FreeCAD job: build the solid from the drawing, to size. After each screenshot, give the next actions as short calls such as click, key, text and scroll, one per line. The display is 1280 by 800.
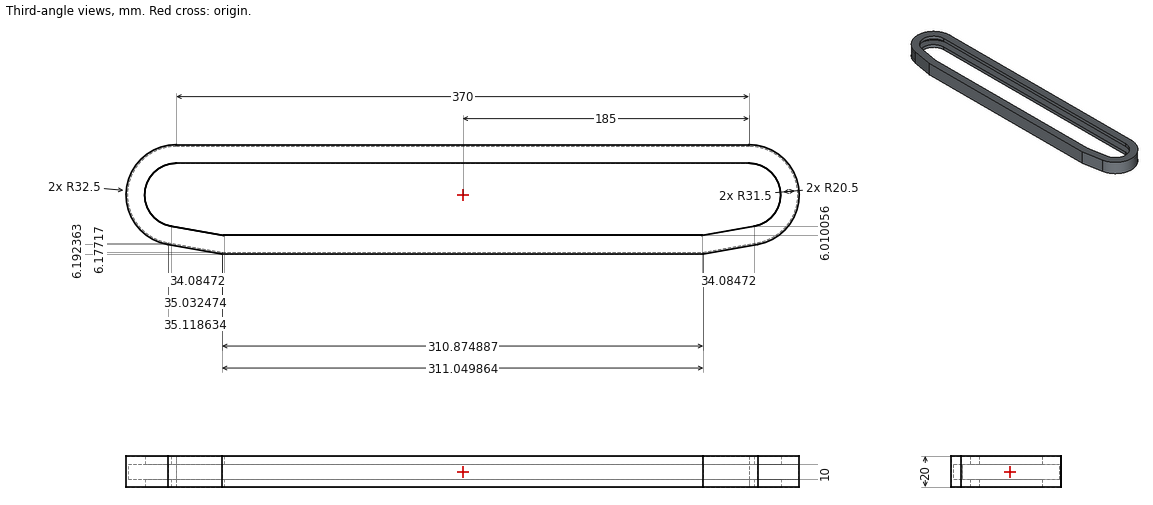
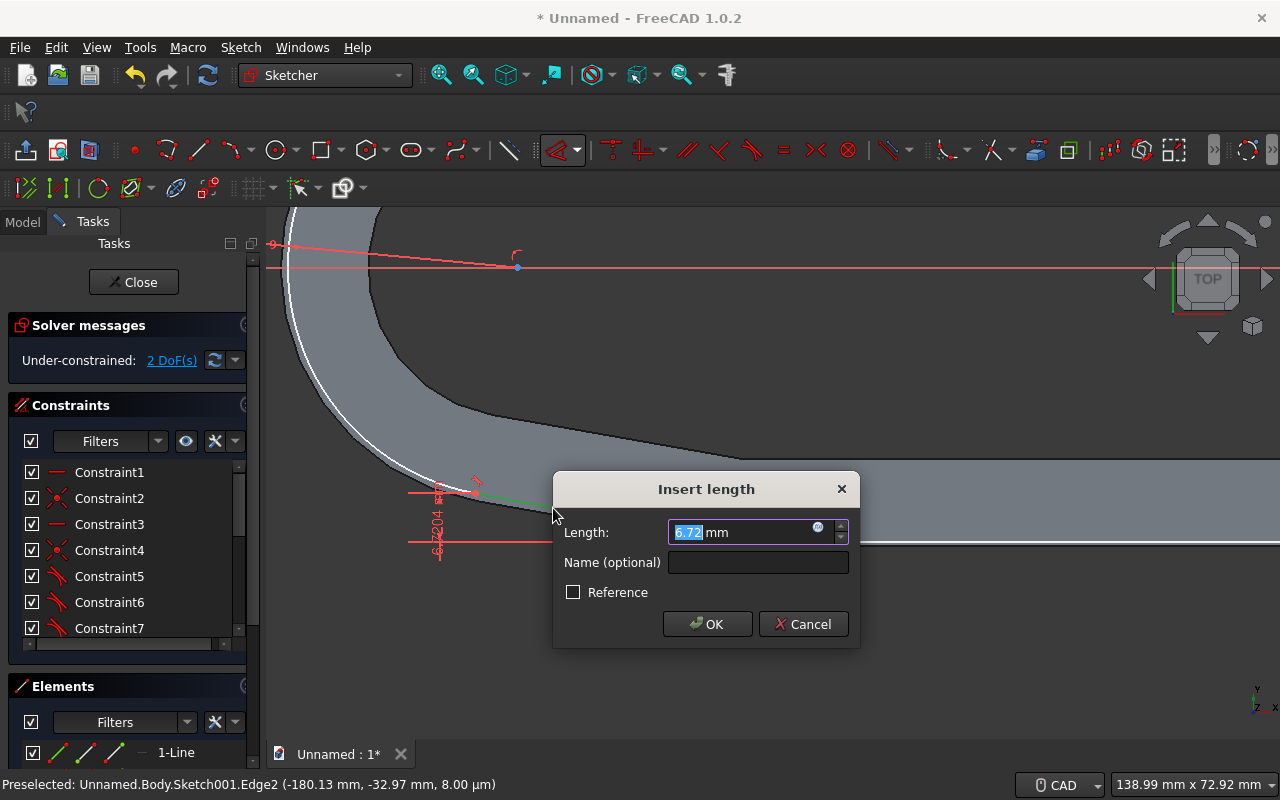
text(6.17717)
key(Return)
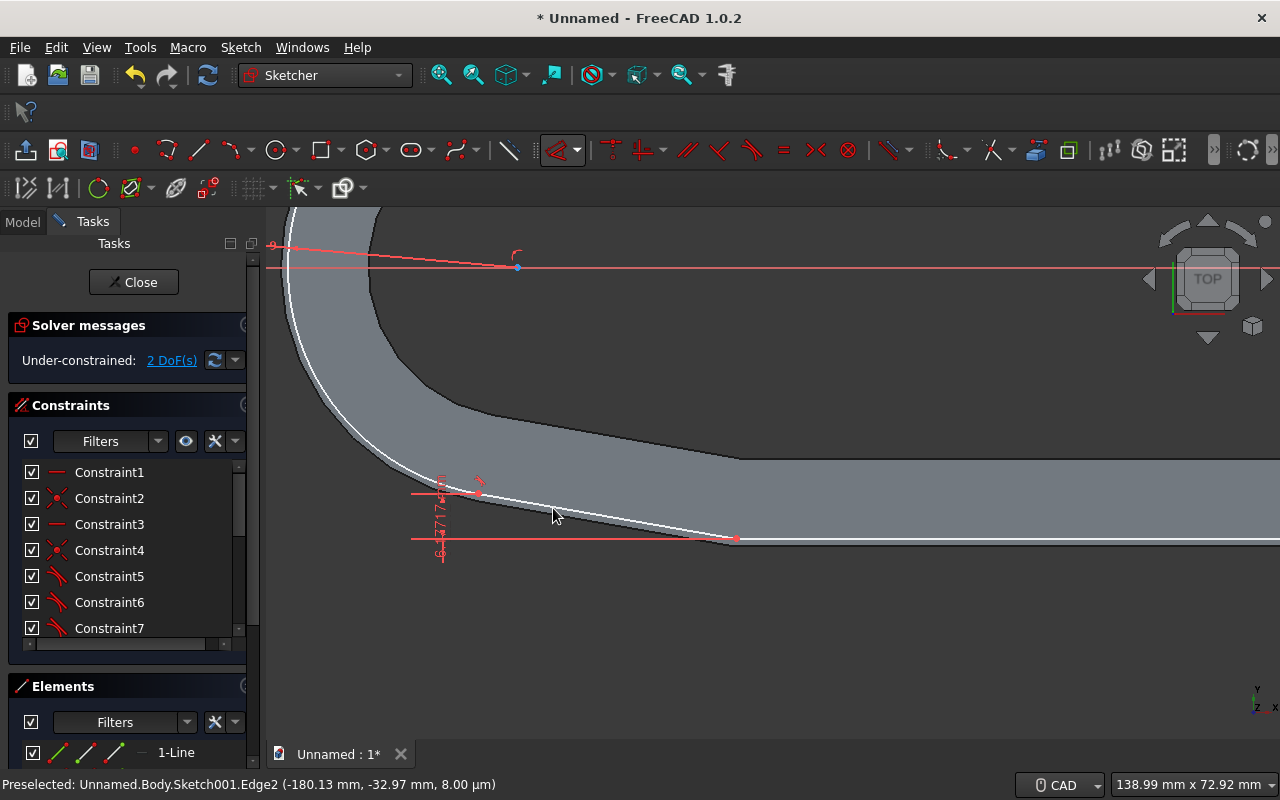
scroll(410, 520, down, 8)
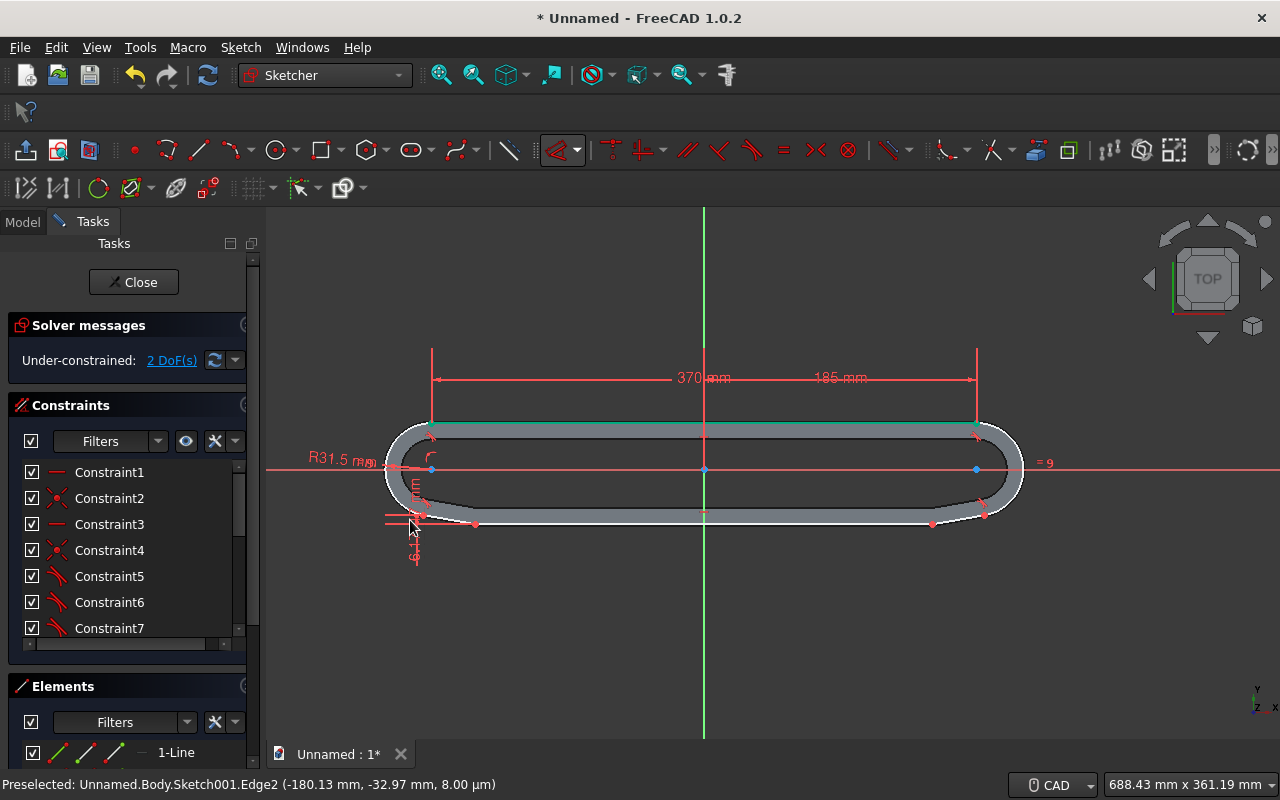
click(613, 524)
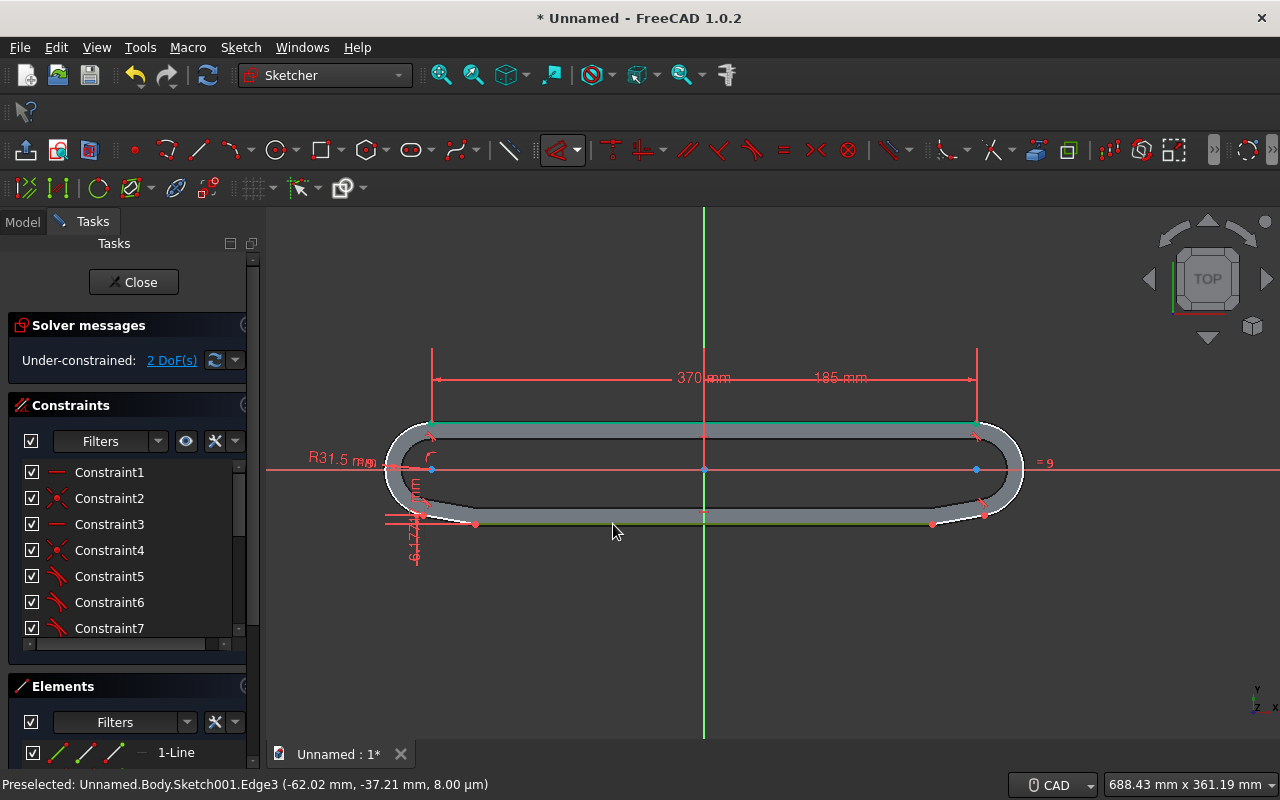
key(l)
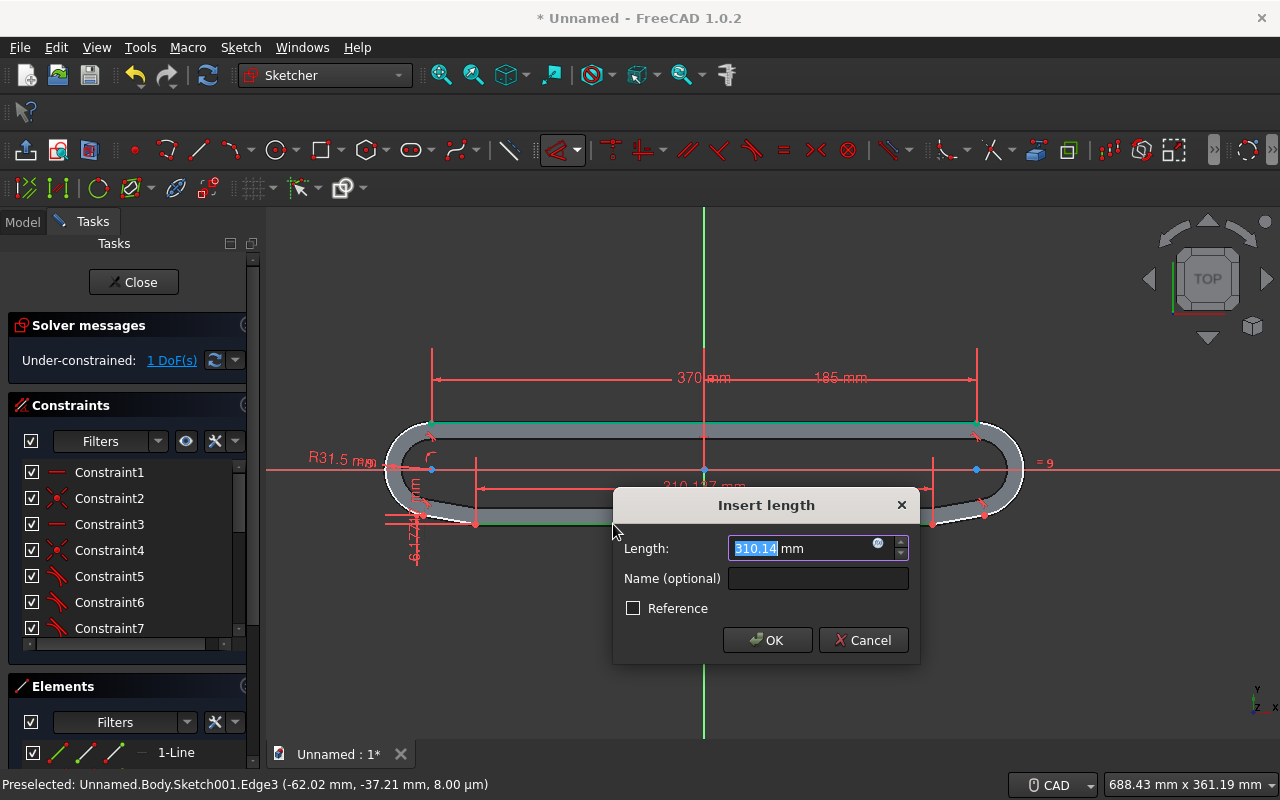
text(310.874887)
key(Return)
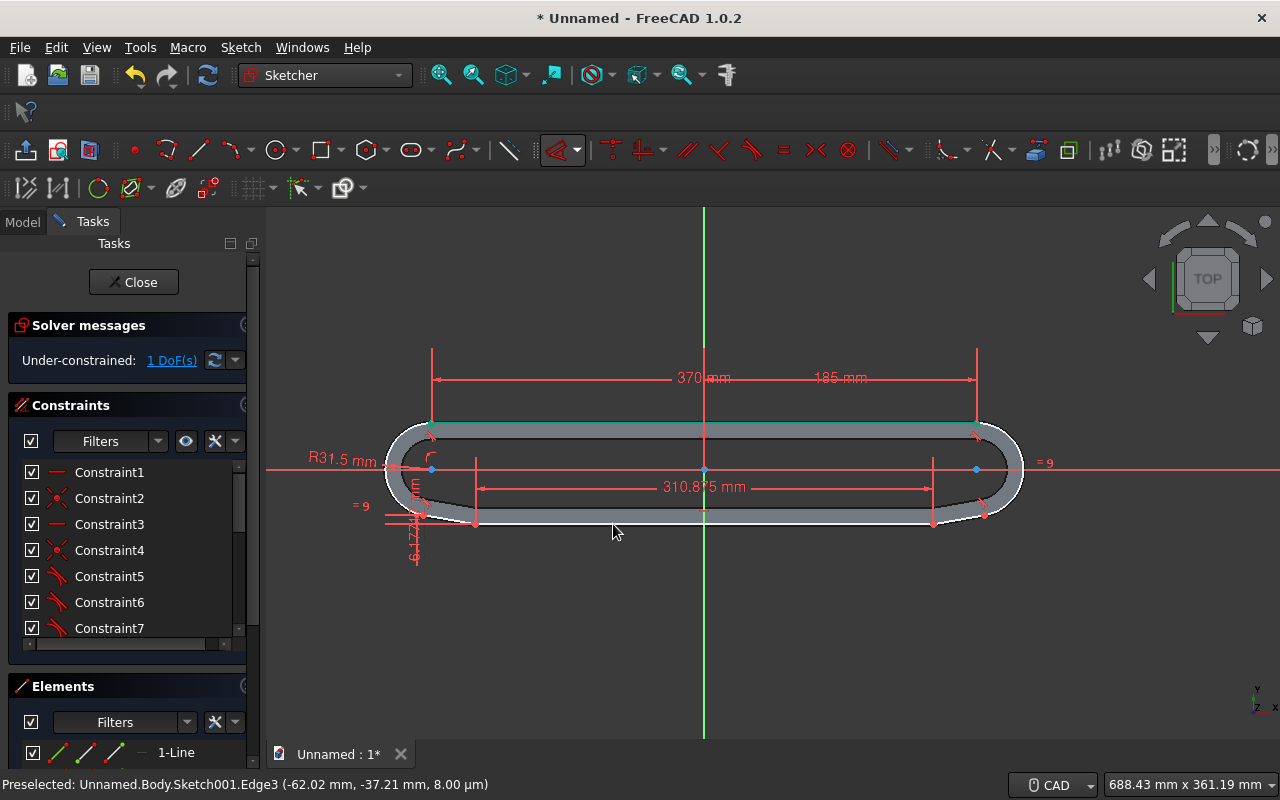
click(439, 518)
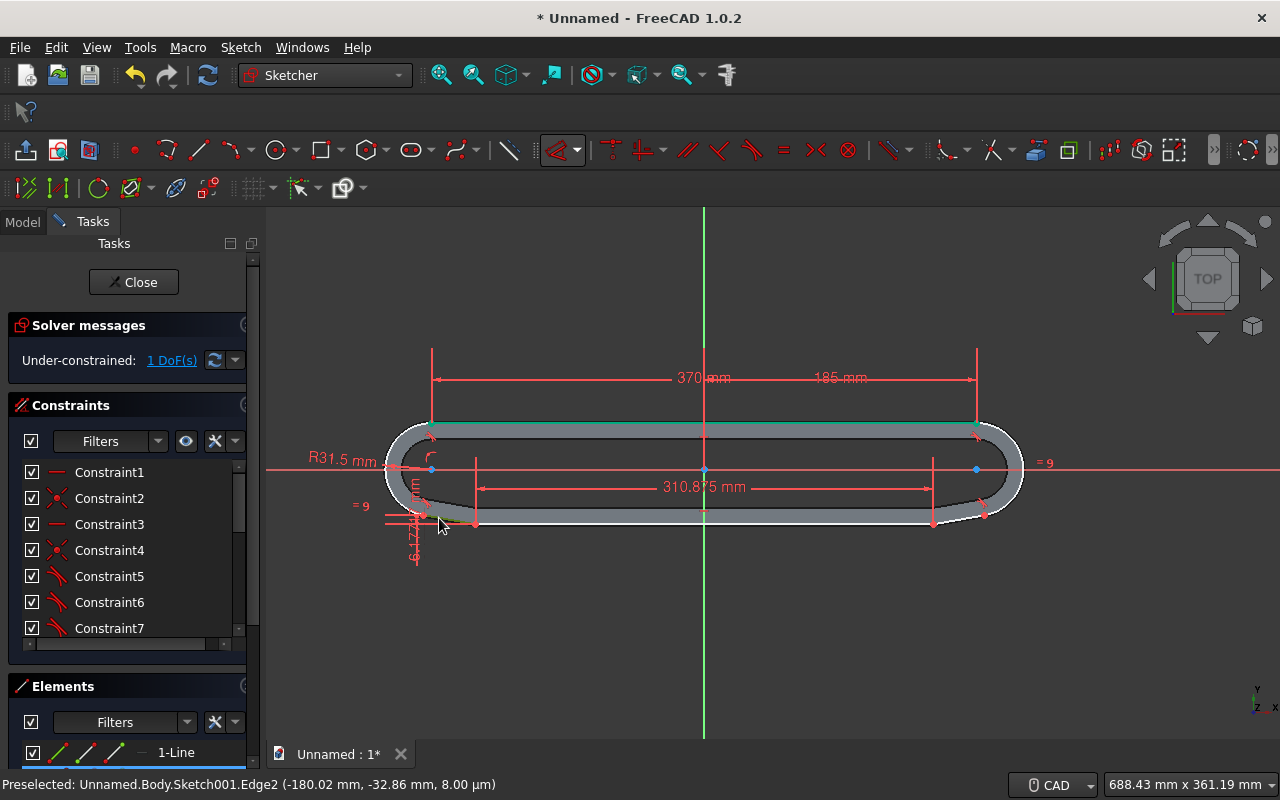
key(l)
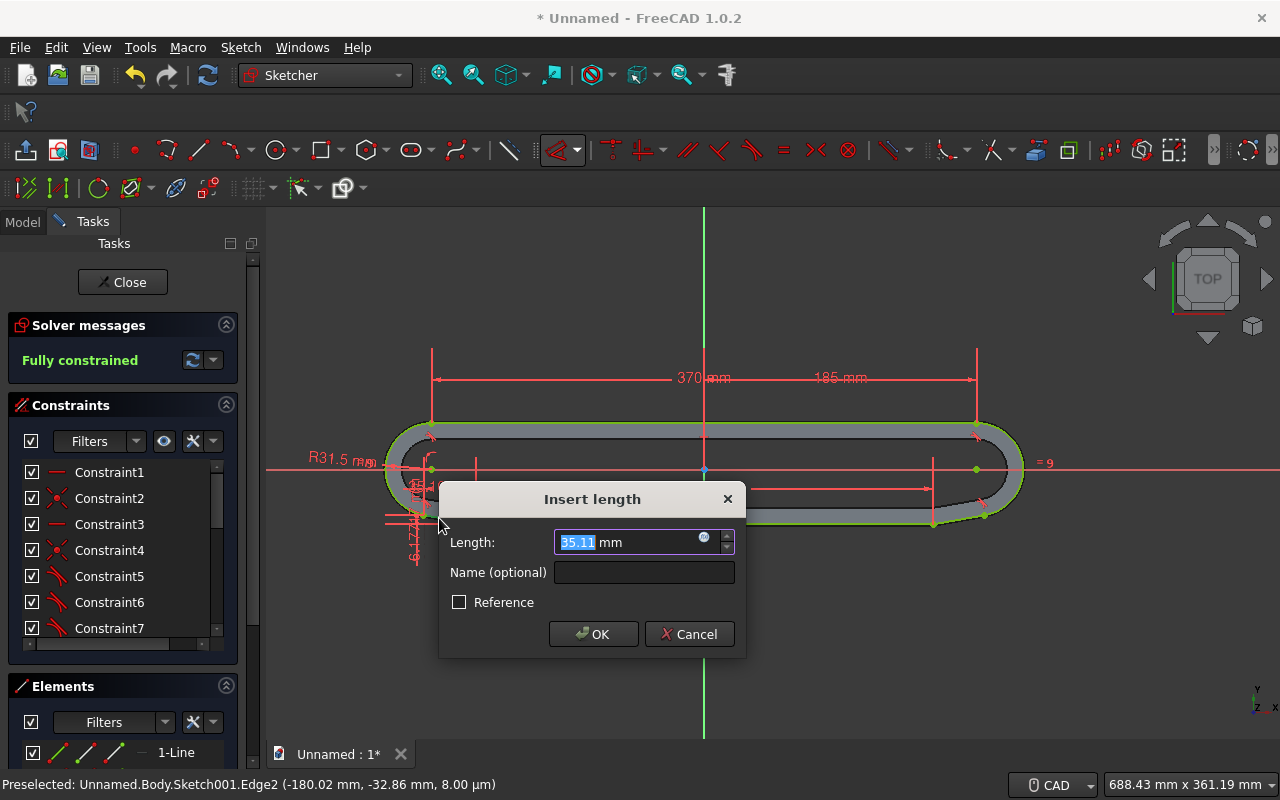
text(35.032474)
key(Return)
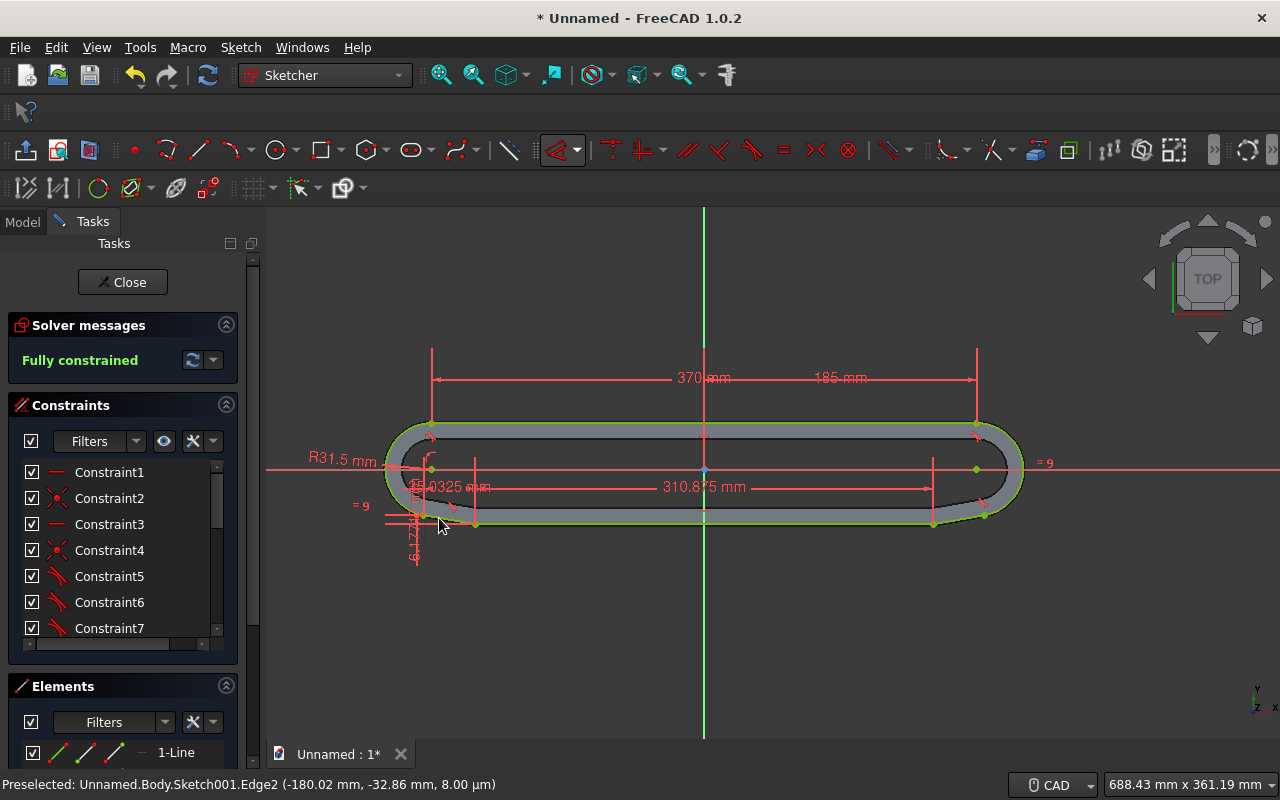
click(123, 282)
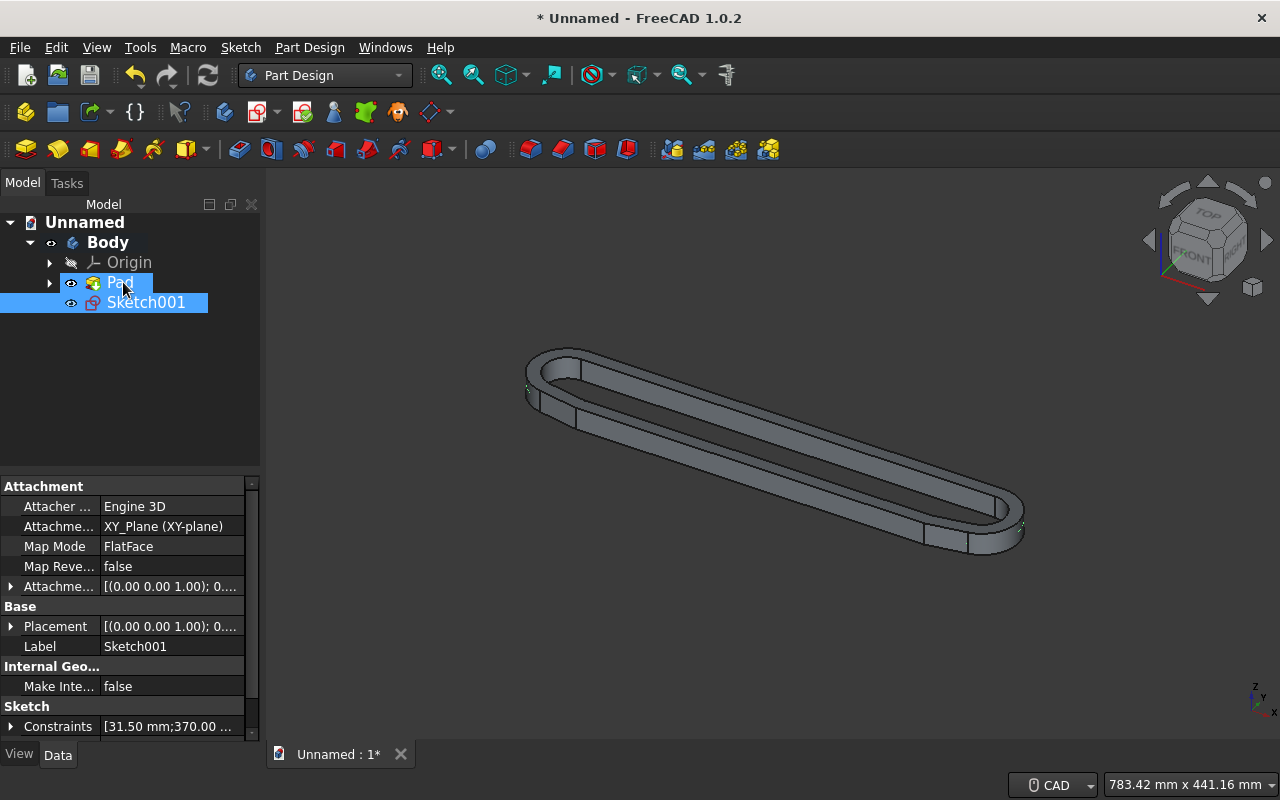
click(240, 150)